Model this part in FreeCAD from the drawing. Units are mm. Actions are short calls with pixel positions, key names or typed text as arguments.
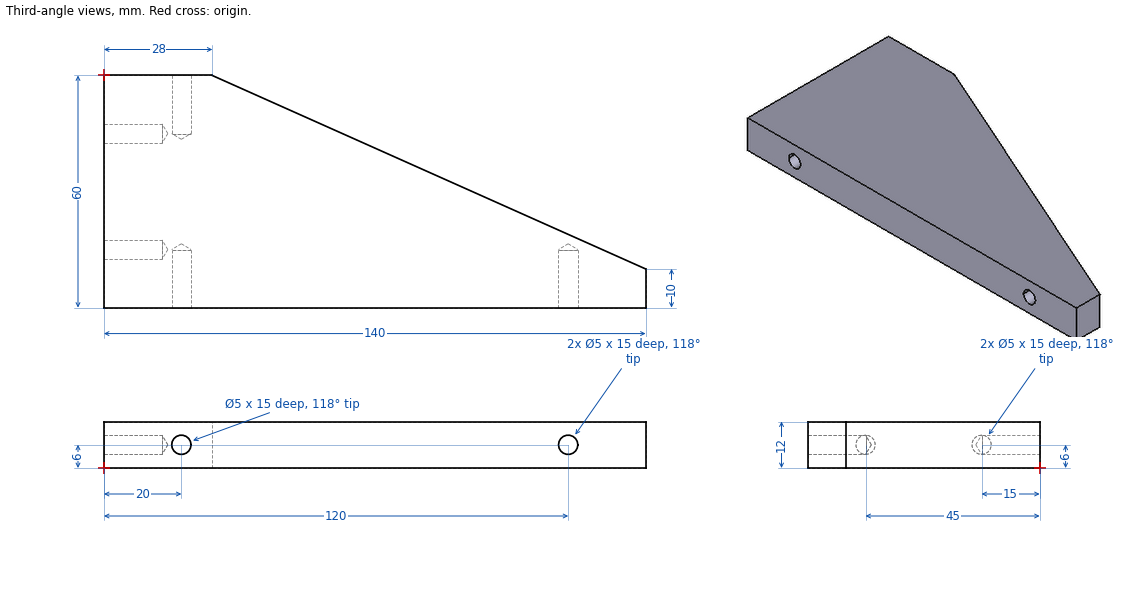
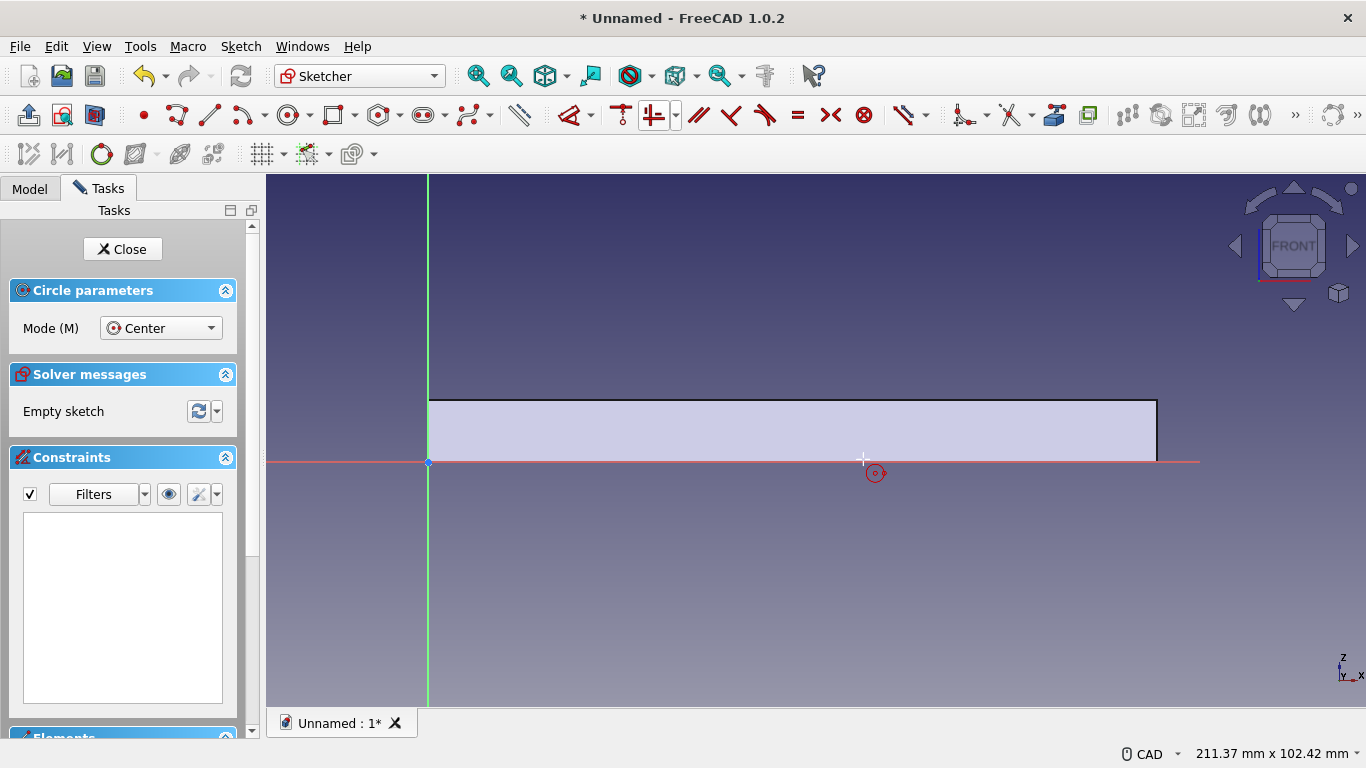
scroll(1053, 431, up, 3)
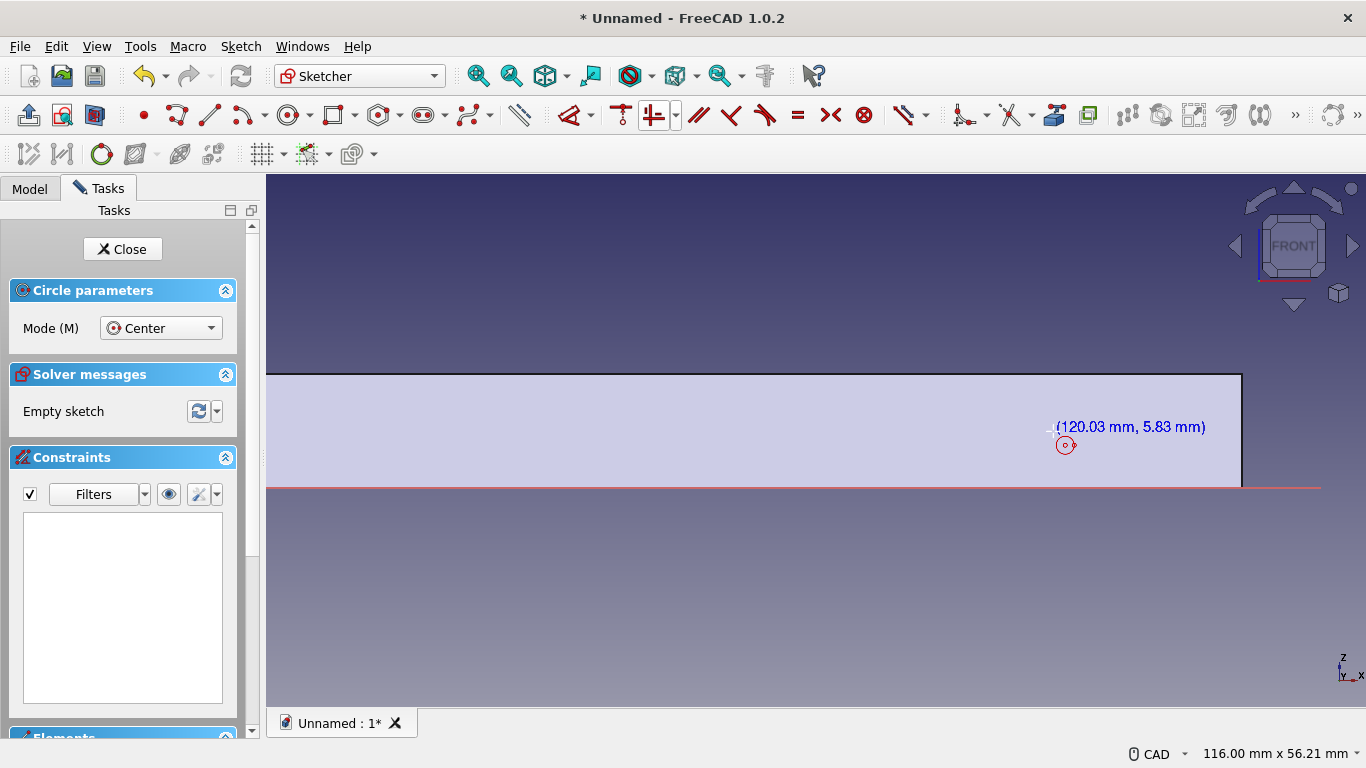
click(1052, 431)
move(1069, 414)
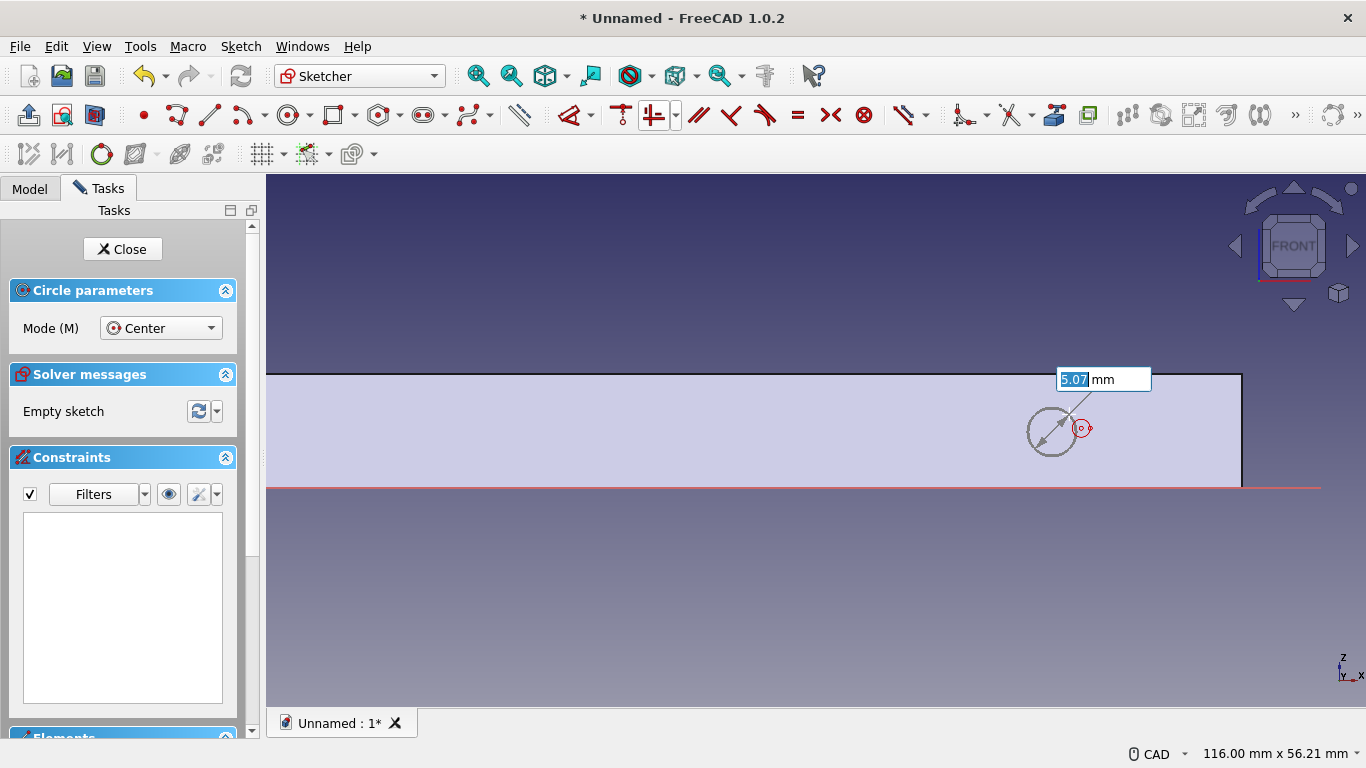
text(5)
key(Return)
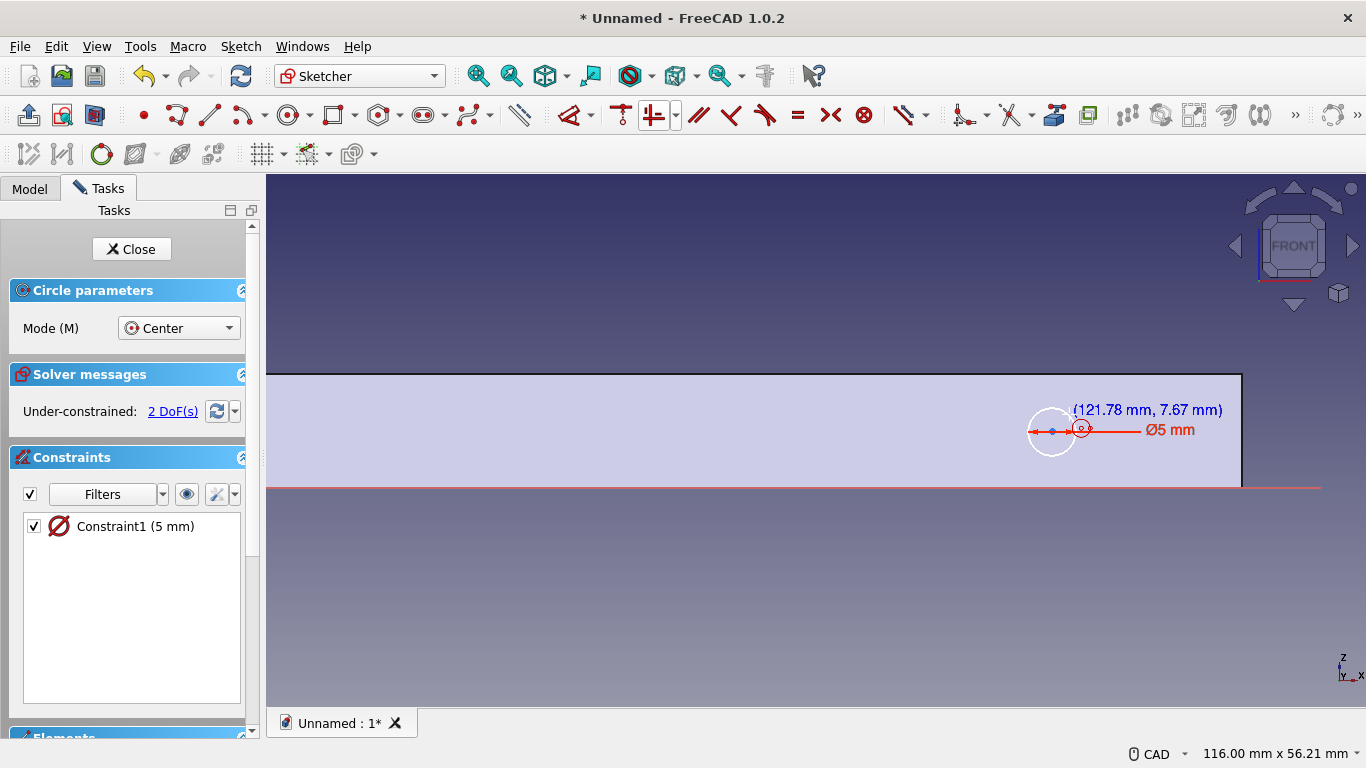
scroll(1055, 432, down, 3)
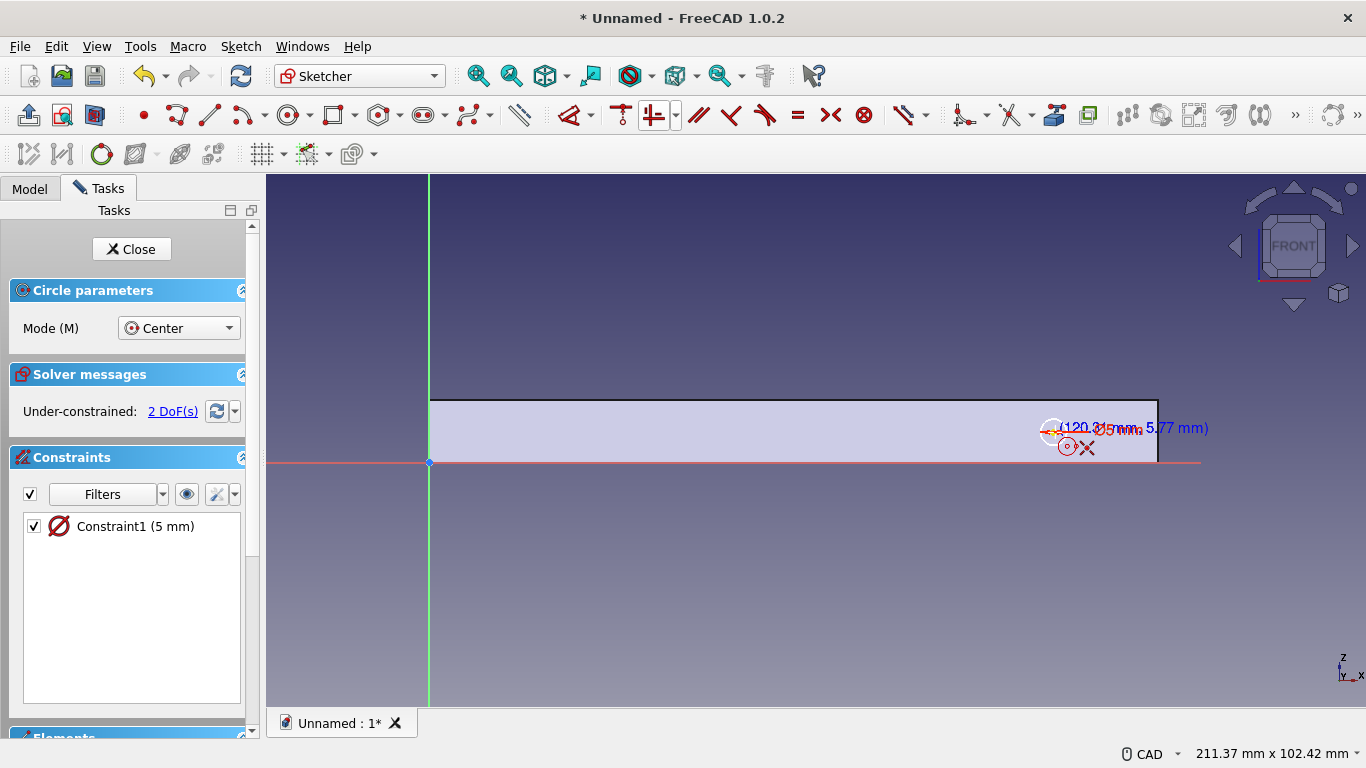
scroll(533, 432, up, 3)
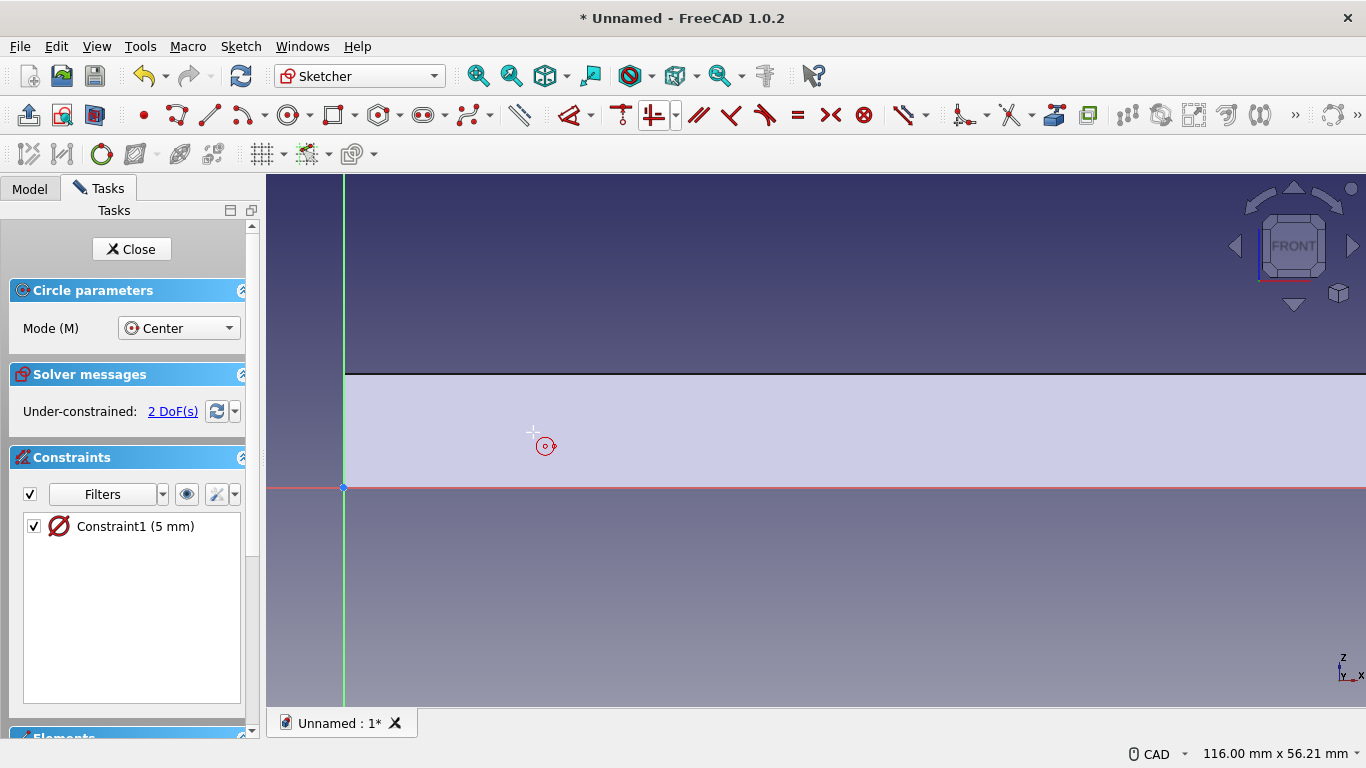
click(533, 431)
move(550, 414)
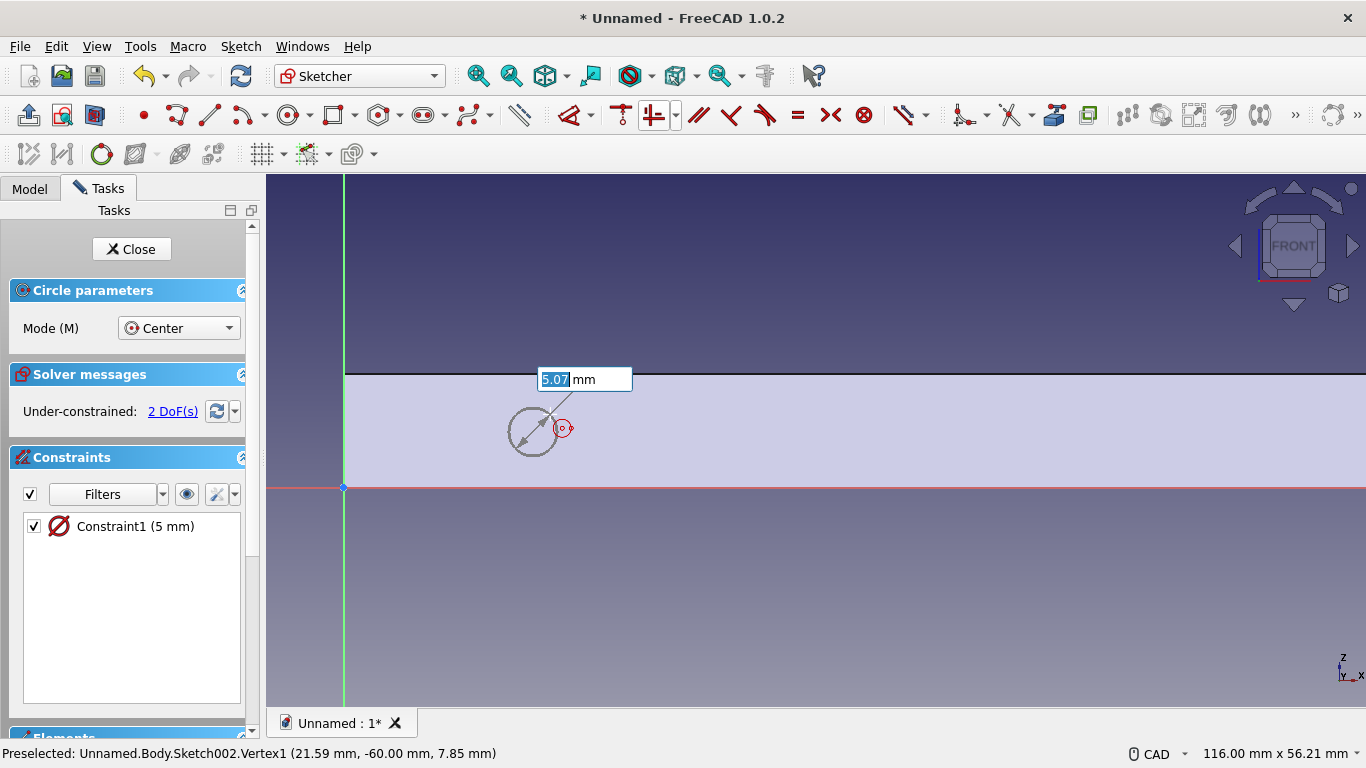
text(5)
key(Return)
key(Escape)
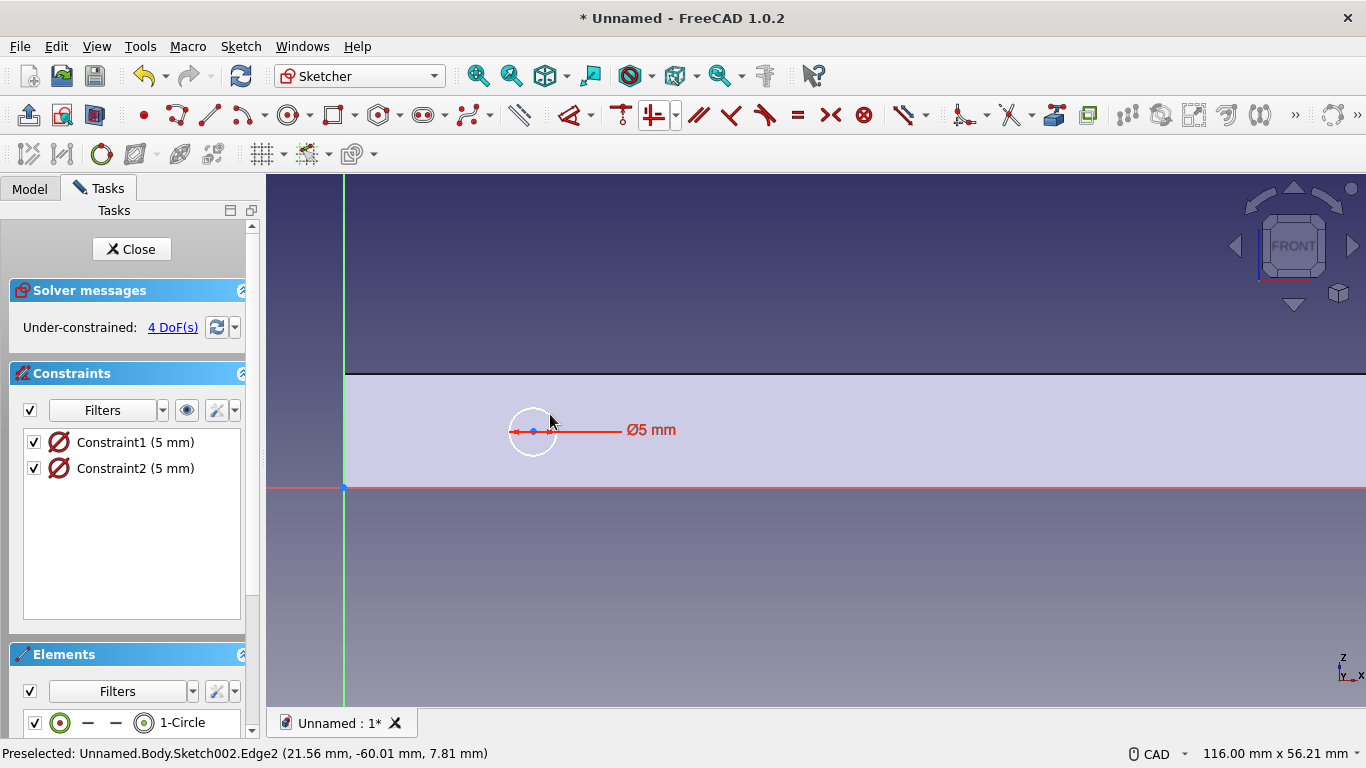
scroll(532, 432, down, 3)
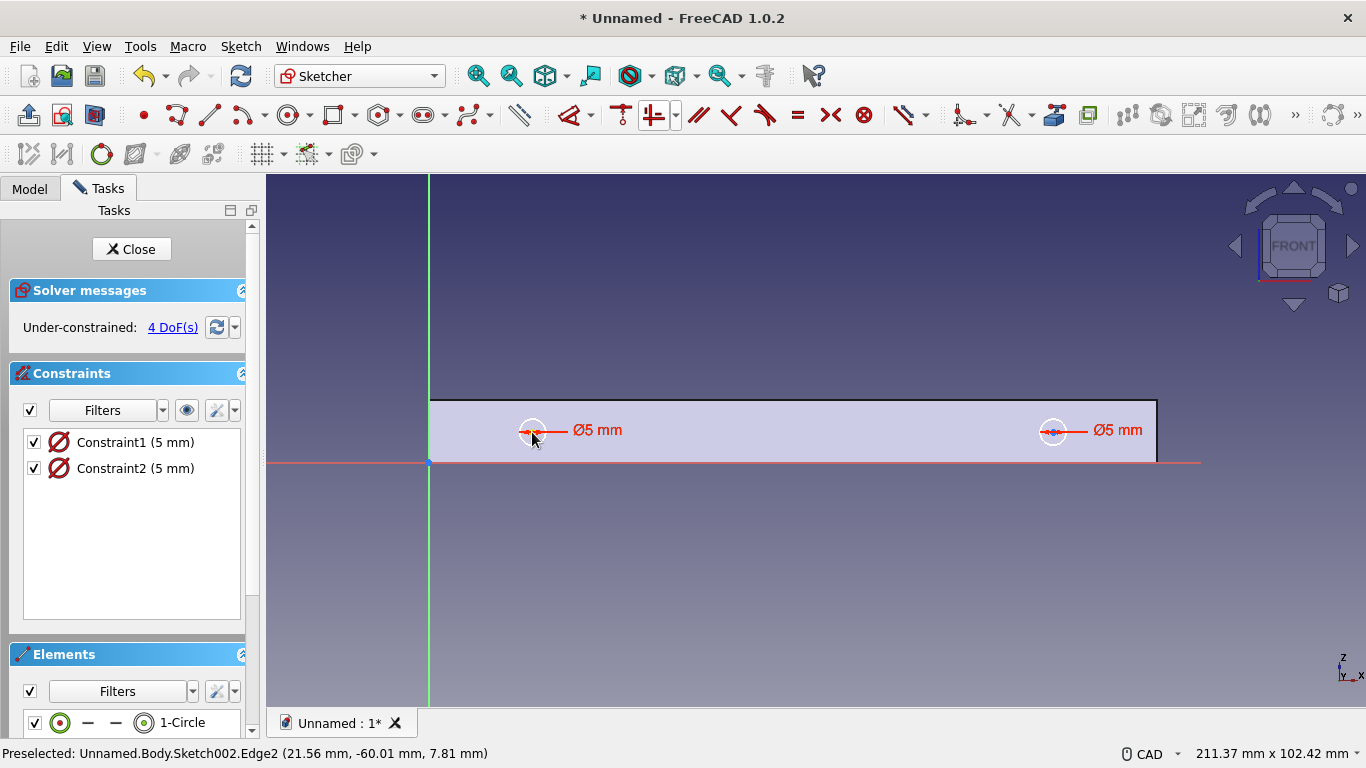
click(1053, 432)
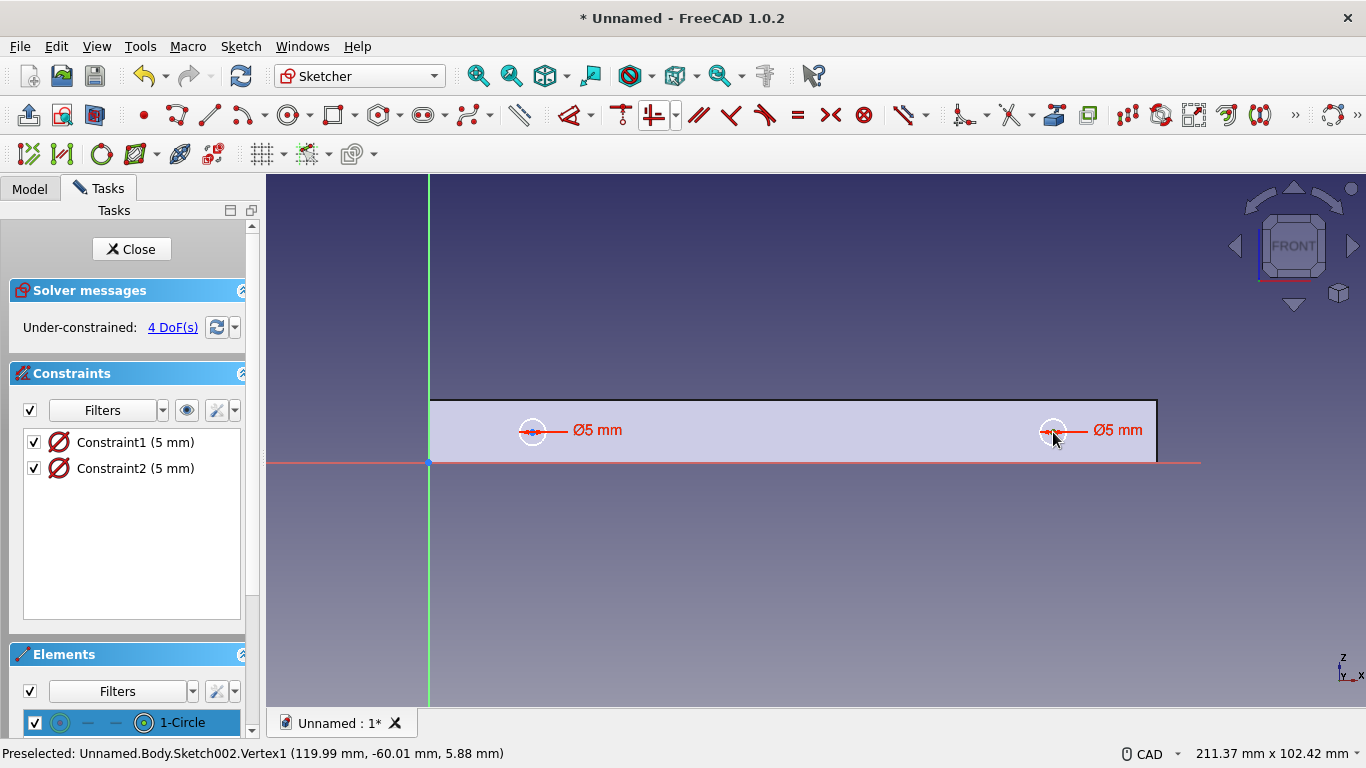
click(533, 432)